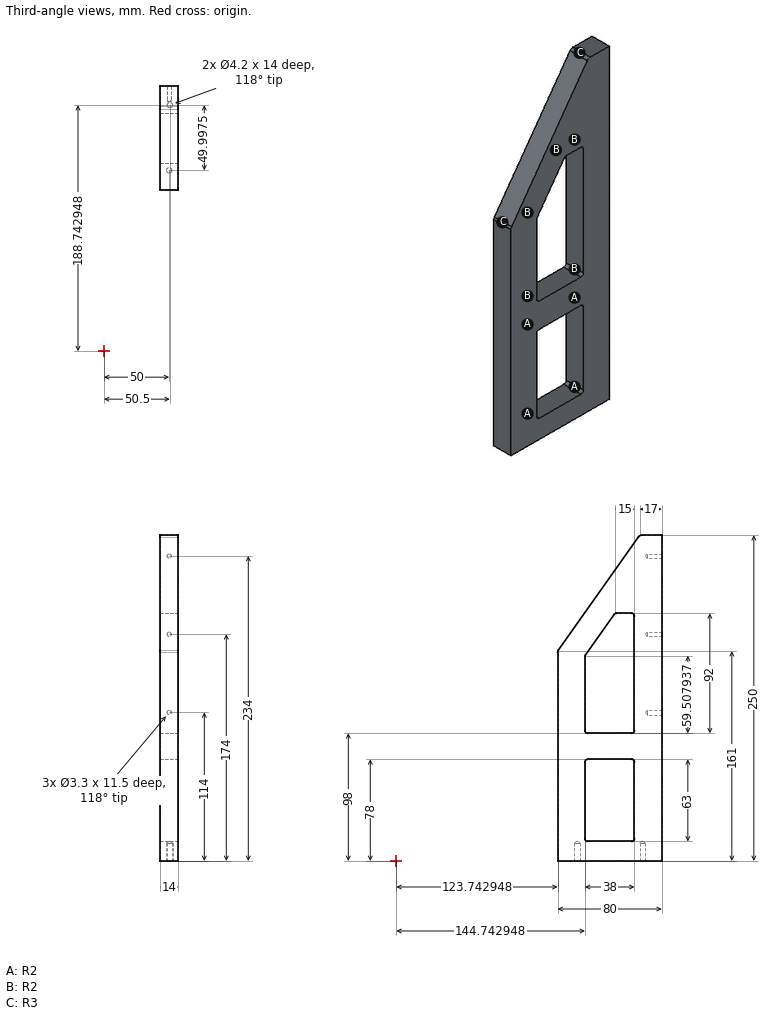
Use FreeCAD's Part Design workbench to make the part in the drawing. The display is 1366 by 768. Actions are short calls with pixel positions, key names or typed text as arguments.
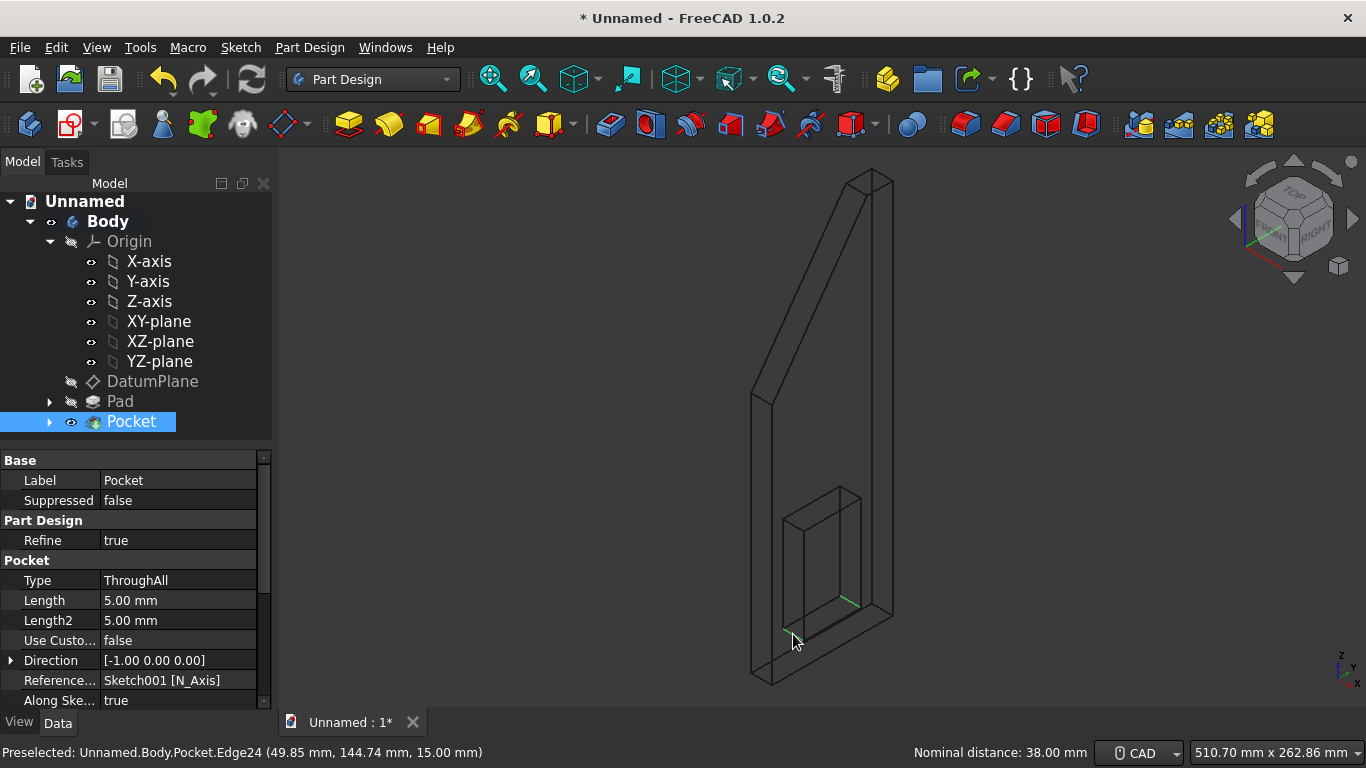
click(793, 524, ctrl)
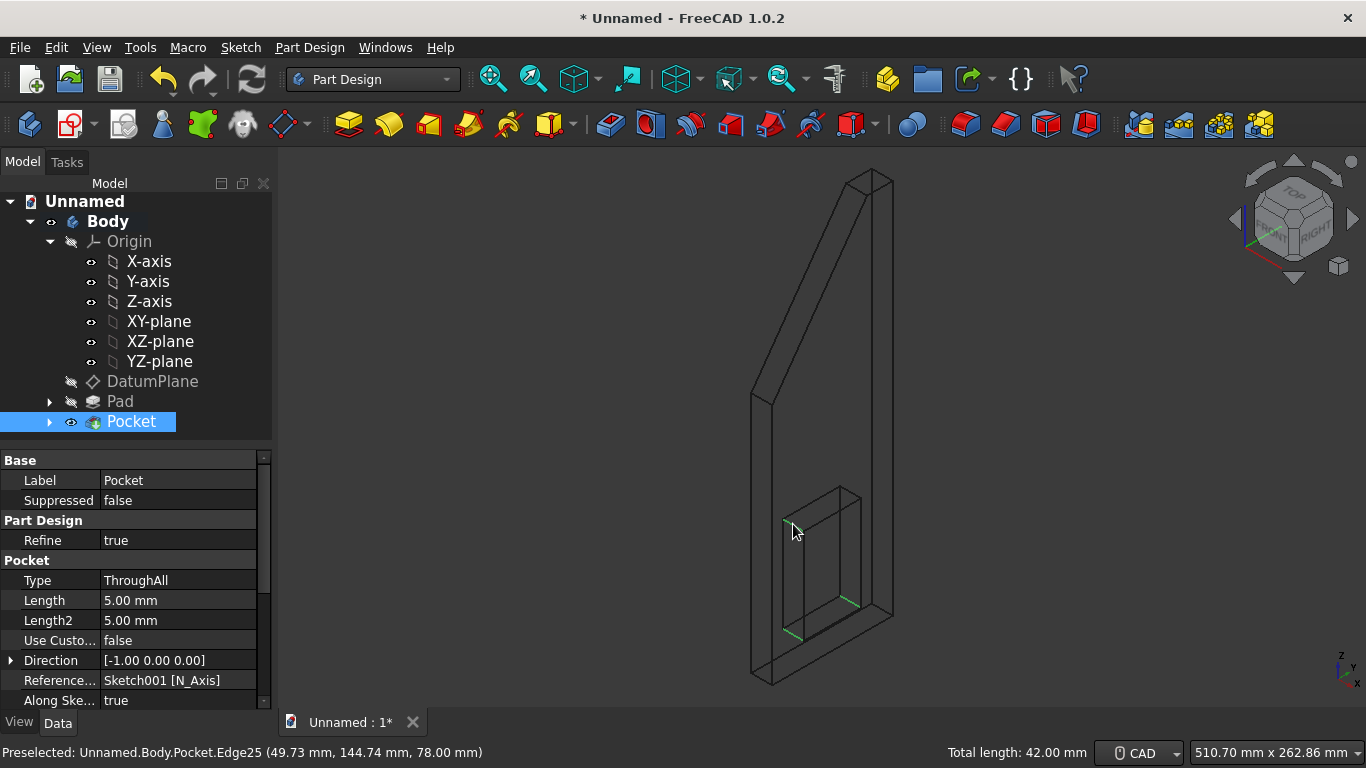
click(851, 491, ctrl)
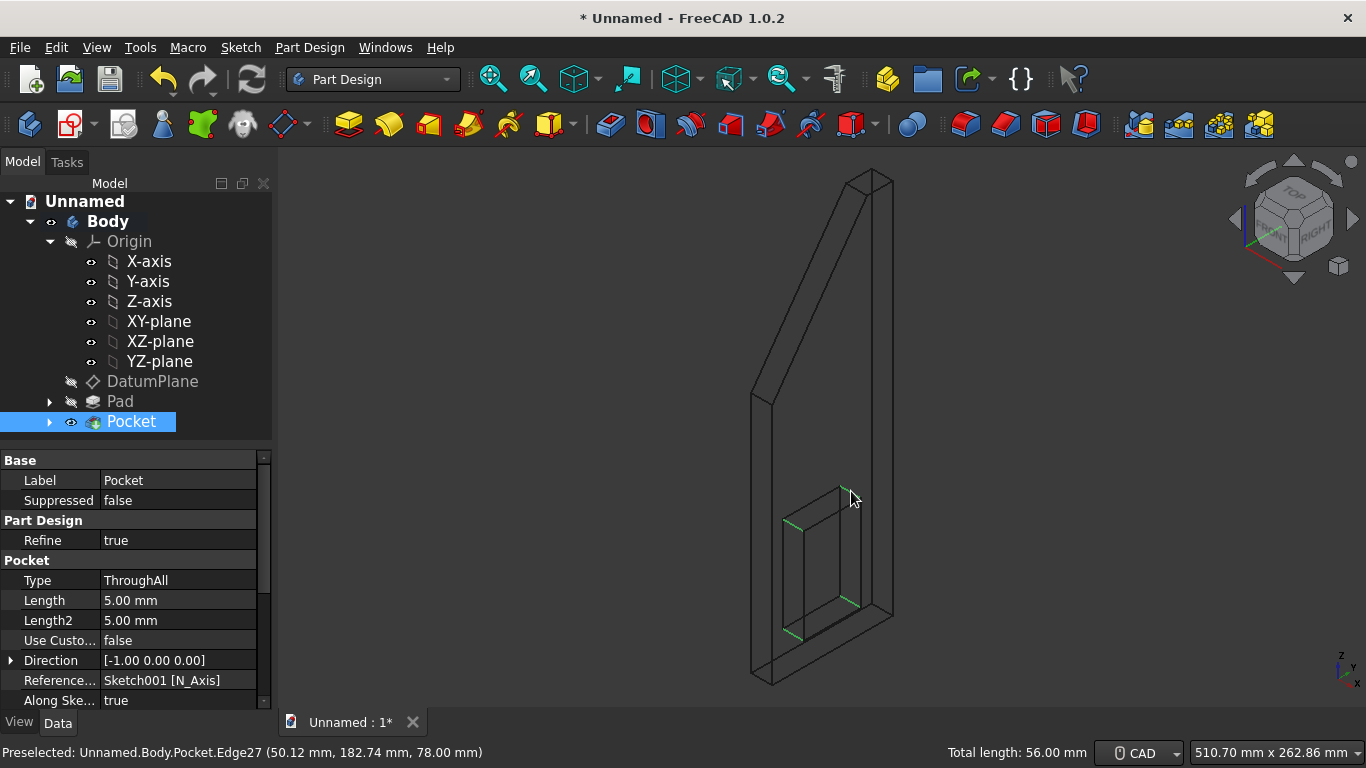
key(v)
key(1)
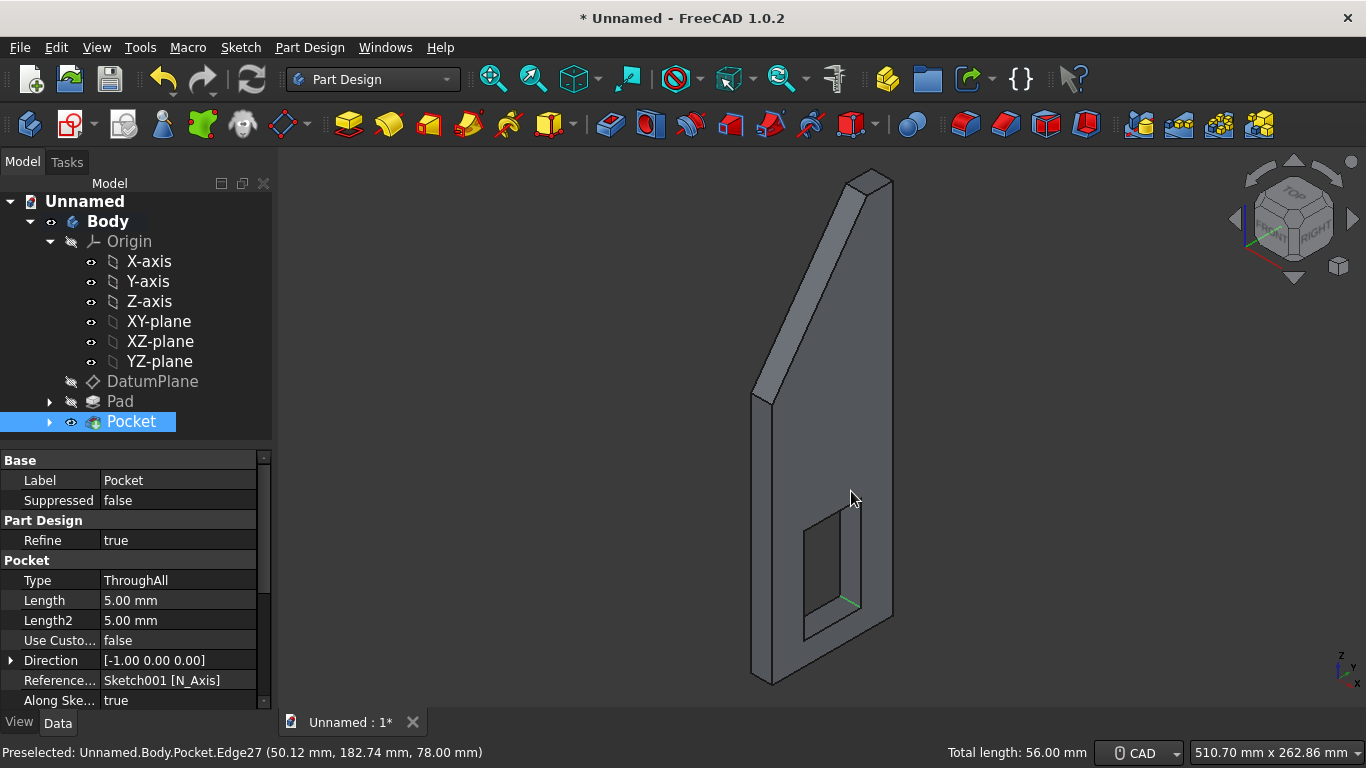
click(966, 124)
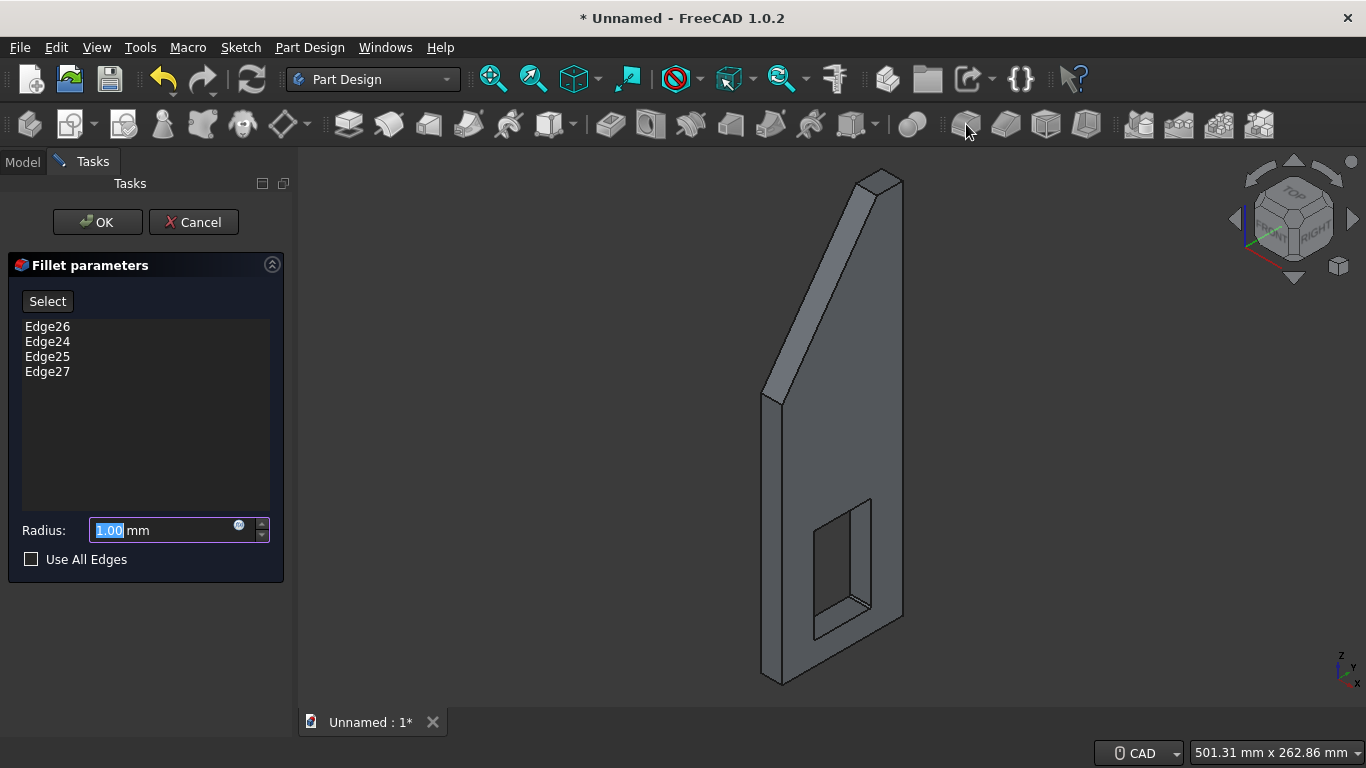
text(2)
key(Tab)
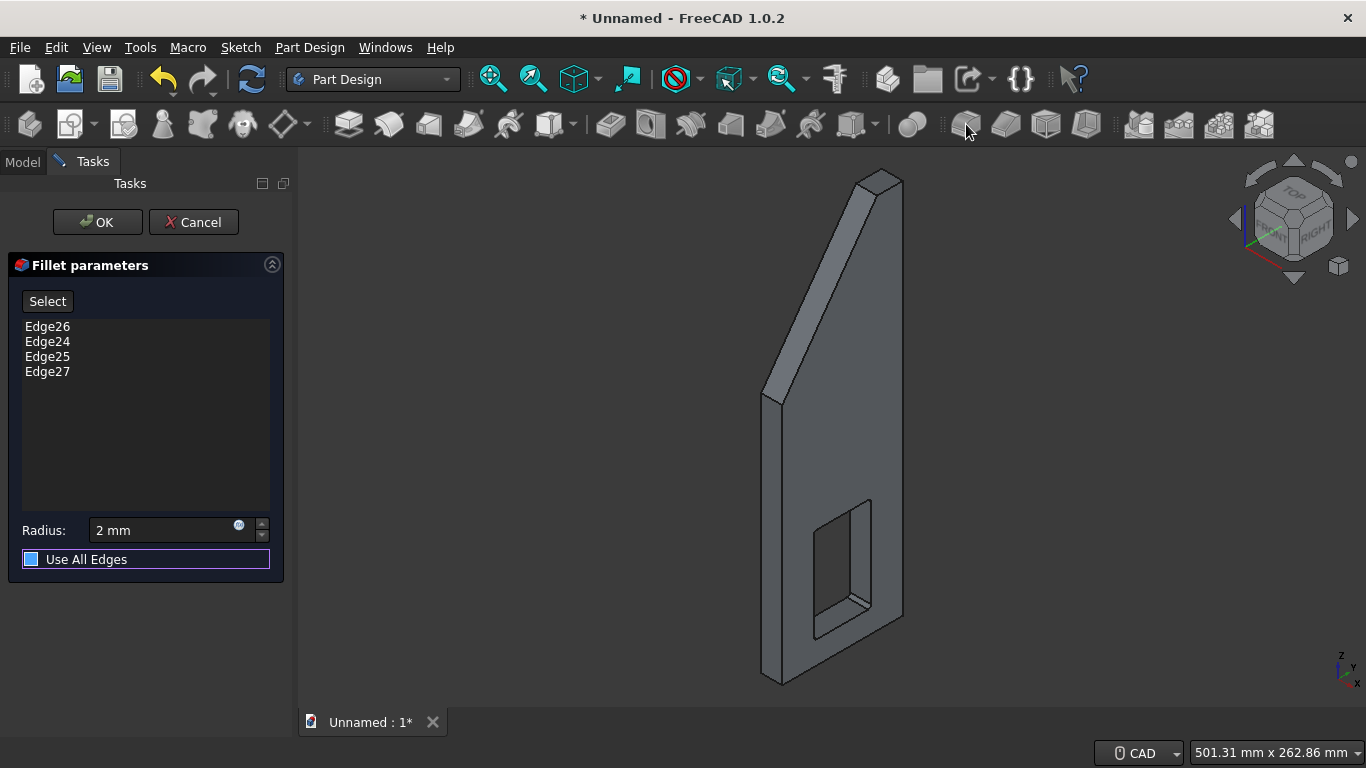
click(98, 222)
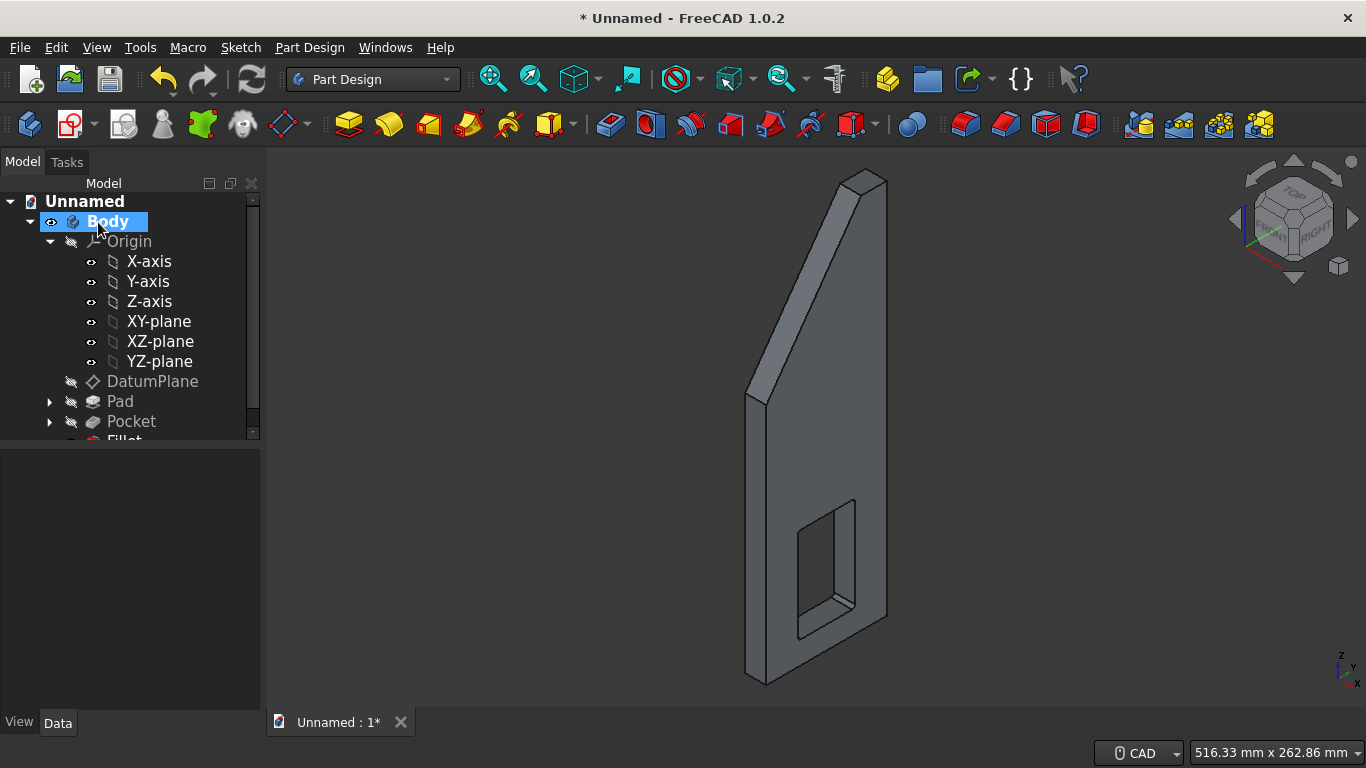
click(827, 432)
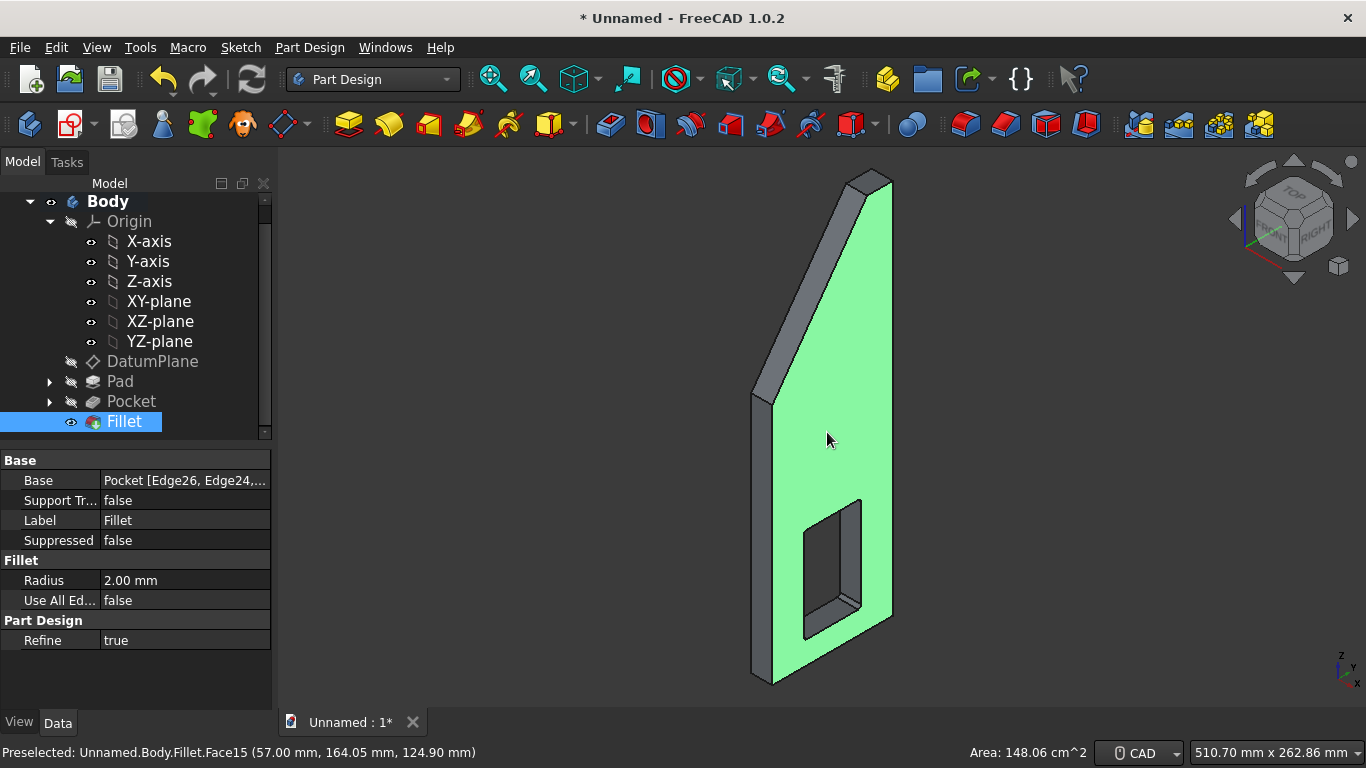
click(70, 124)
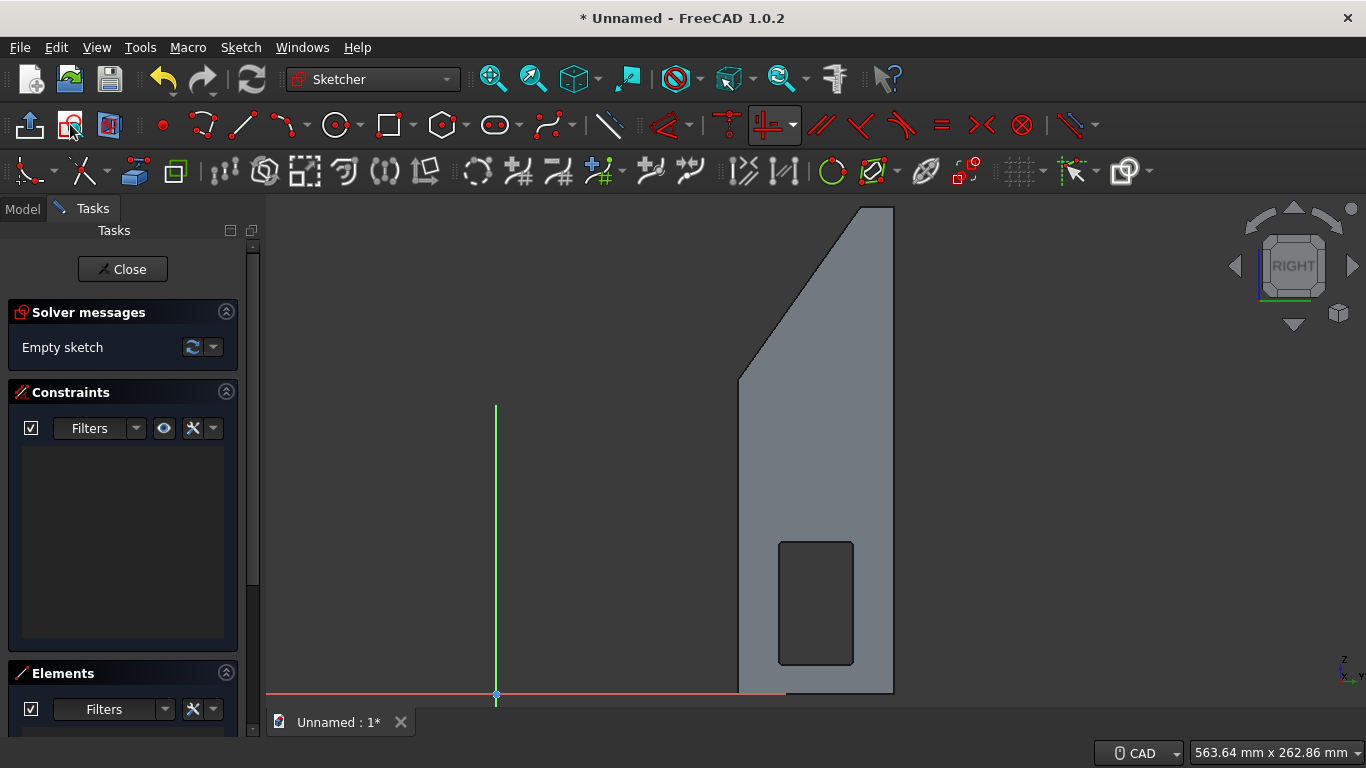
scroll(1076, 222, down, 1)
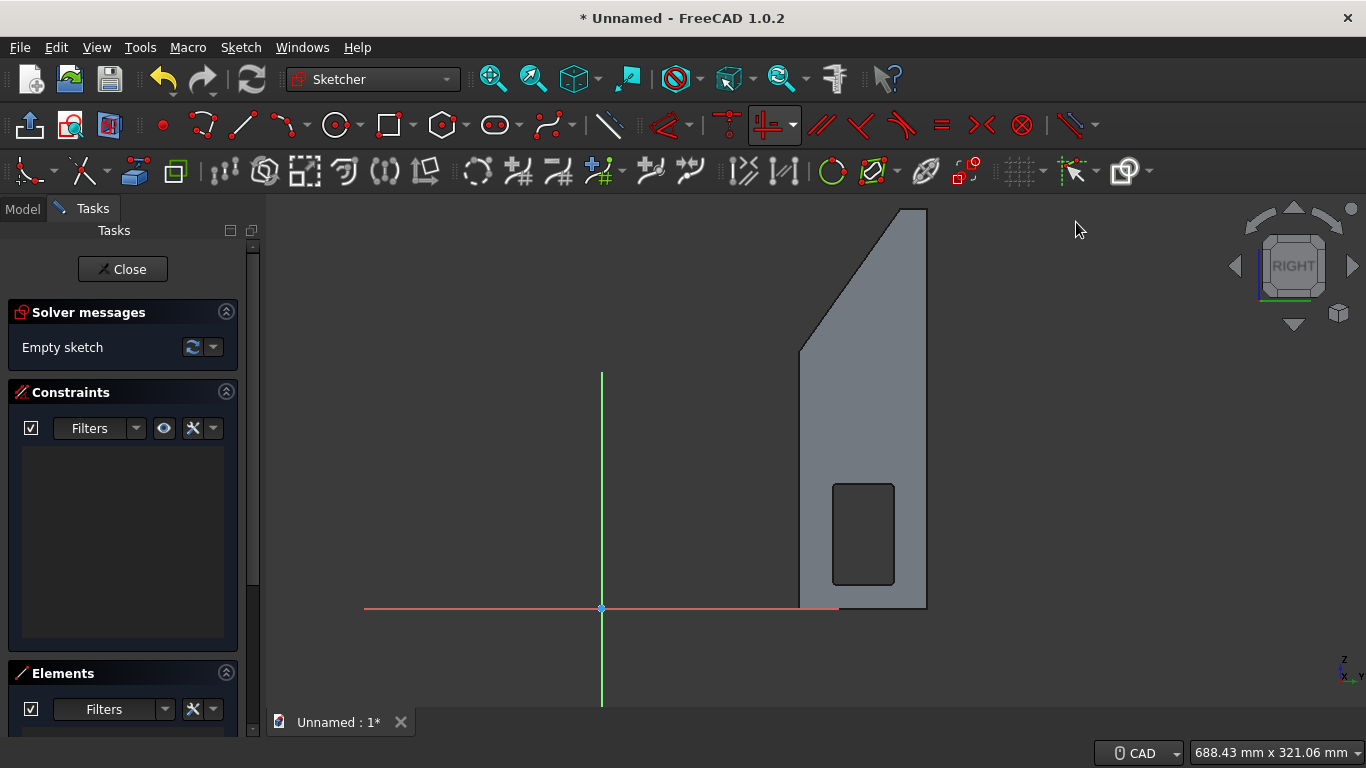
click(204, 126)